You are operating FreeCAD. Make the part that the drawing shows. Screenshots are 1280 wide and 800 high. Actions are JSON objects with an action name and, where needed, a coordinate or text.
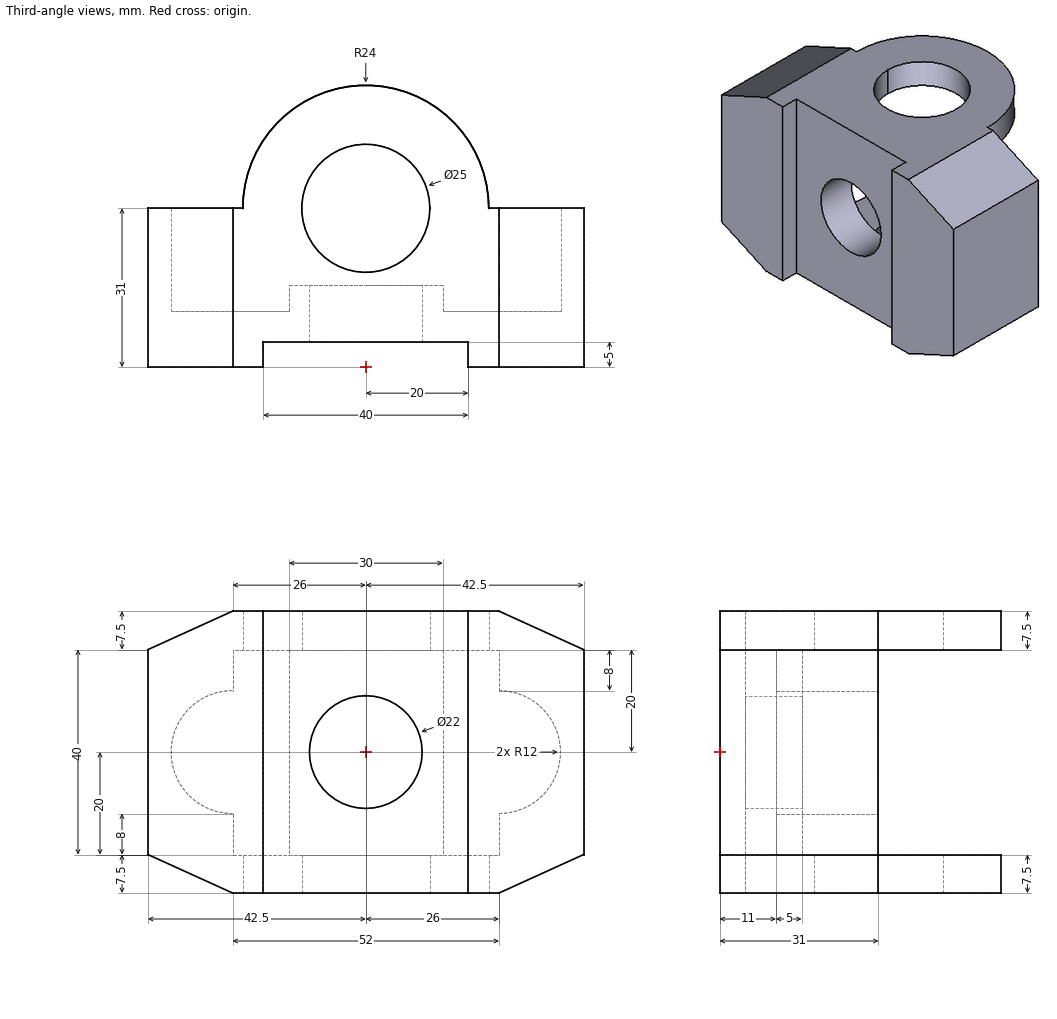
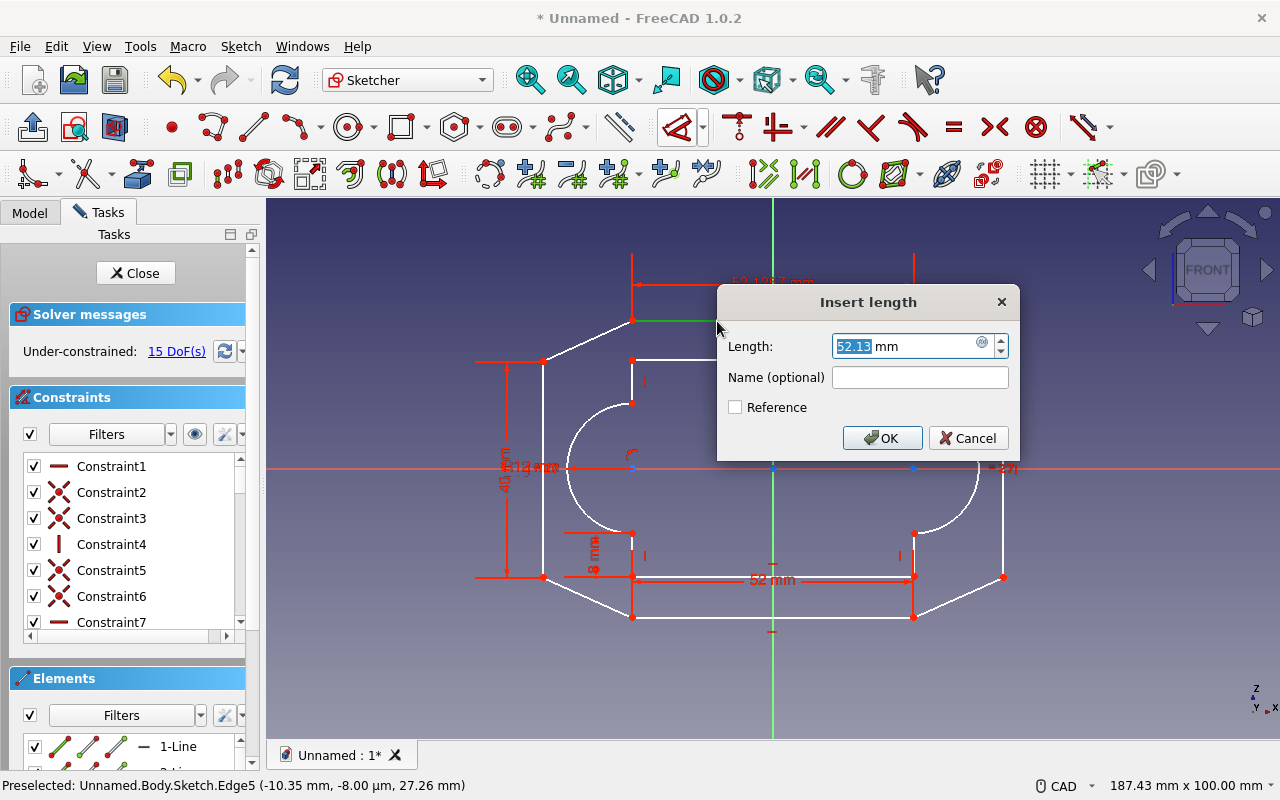
{"action": "type", "text": "52"}
{"action": "key", "text": "Return"}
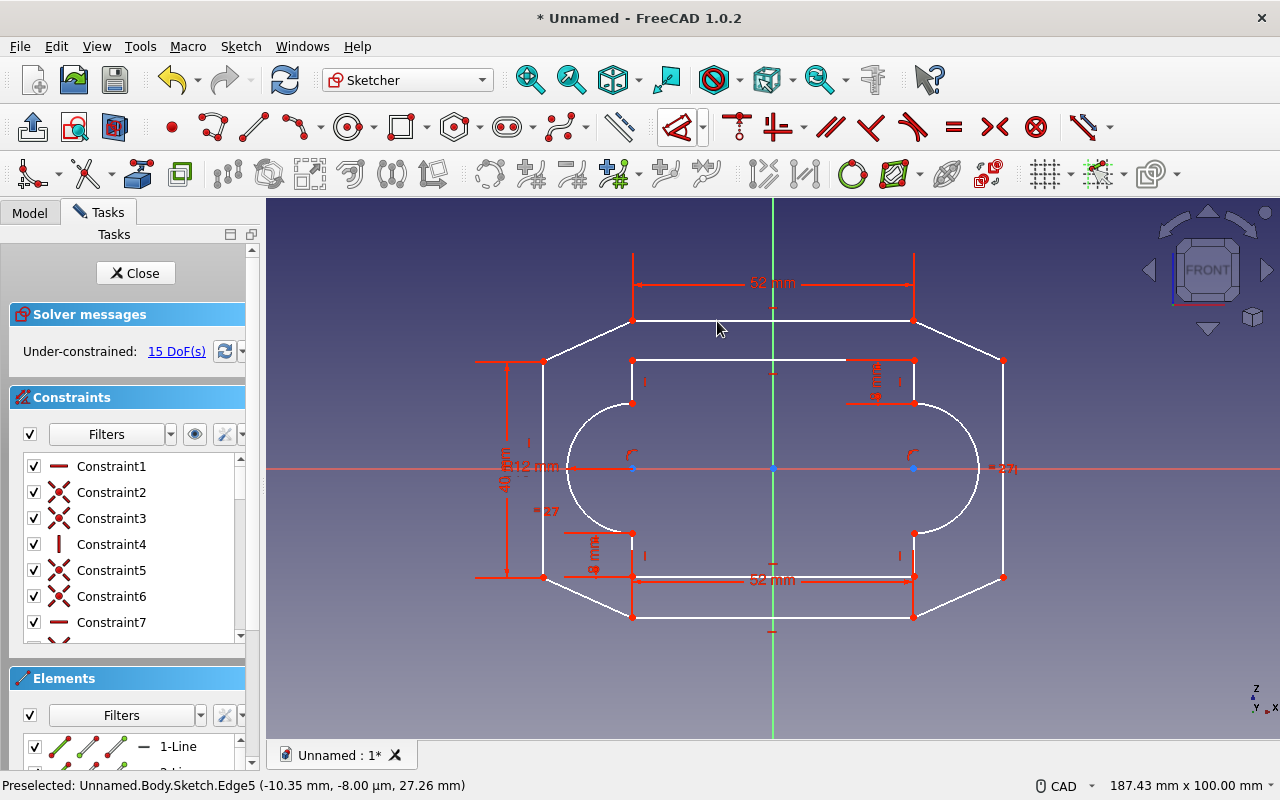
{"action": "left_click", "coordinate": [1003, 426]}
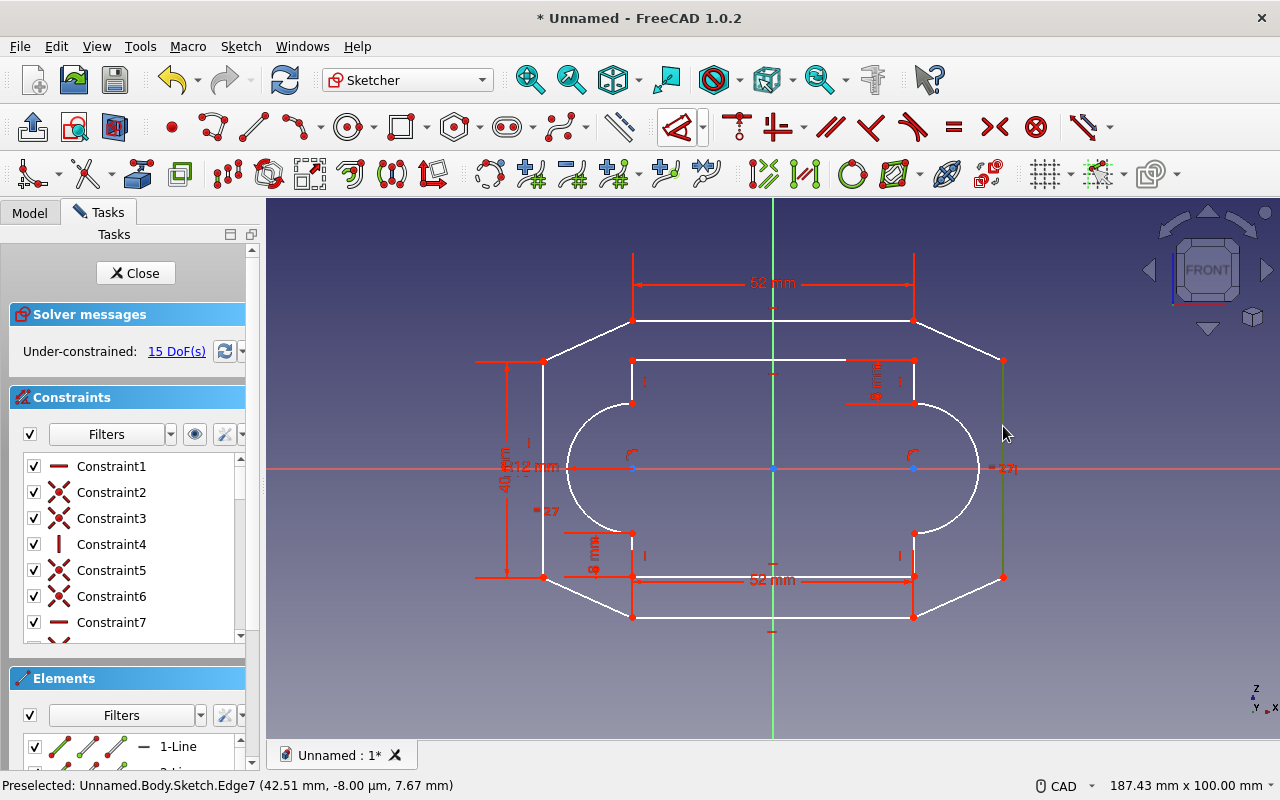
{"action": "key", "text": "i"}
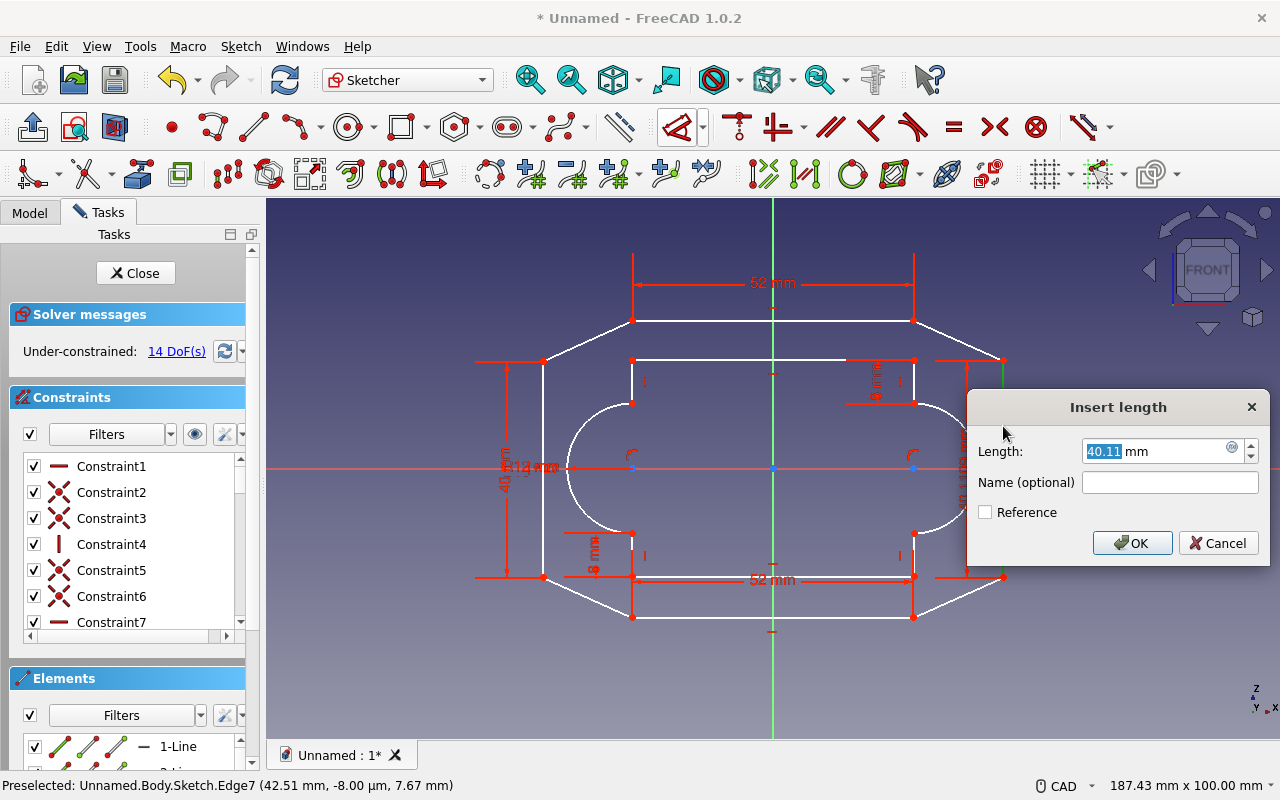
{"action": "type", "text": "40"}
{"action": "key", "text": "Return"}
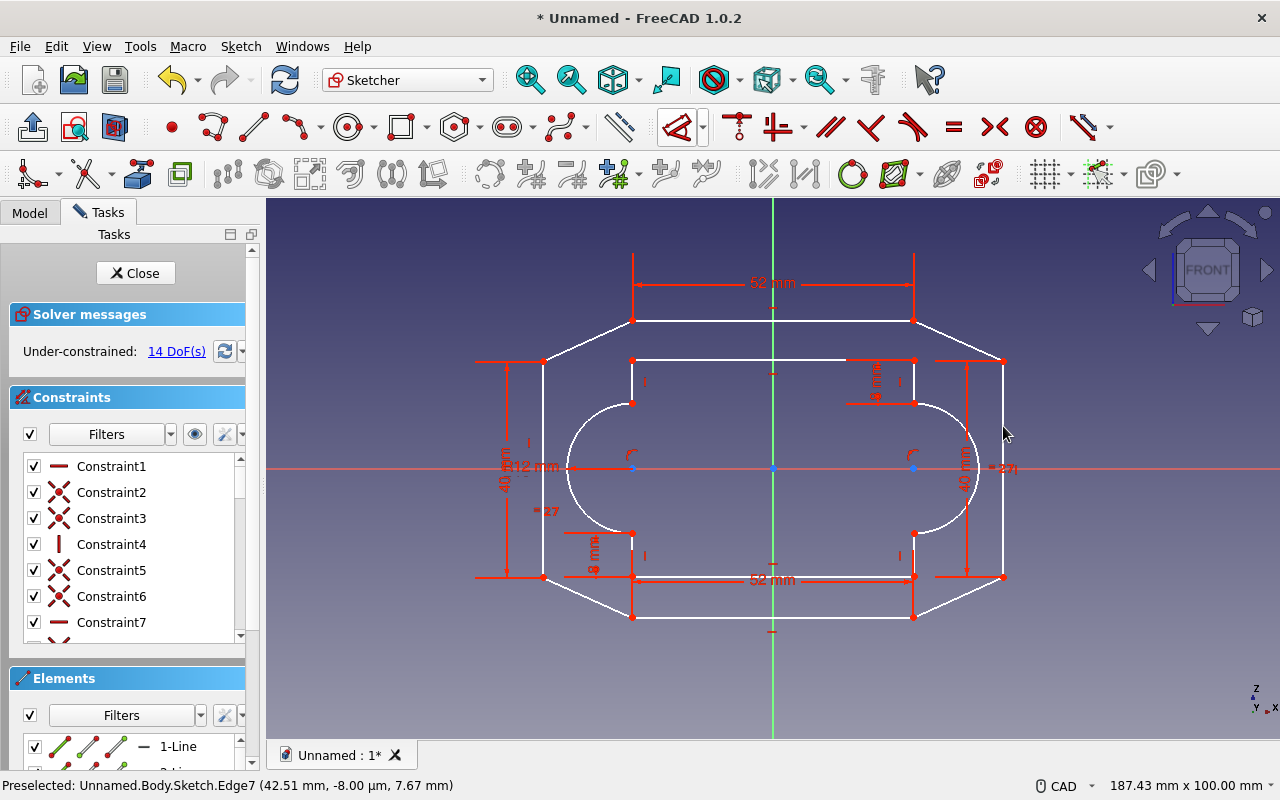
{"action": "left_click", "coordinate": [829, 360]}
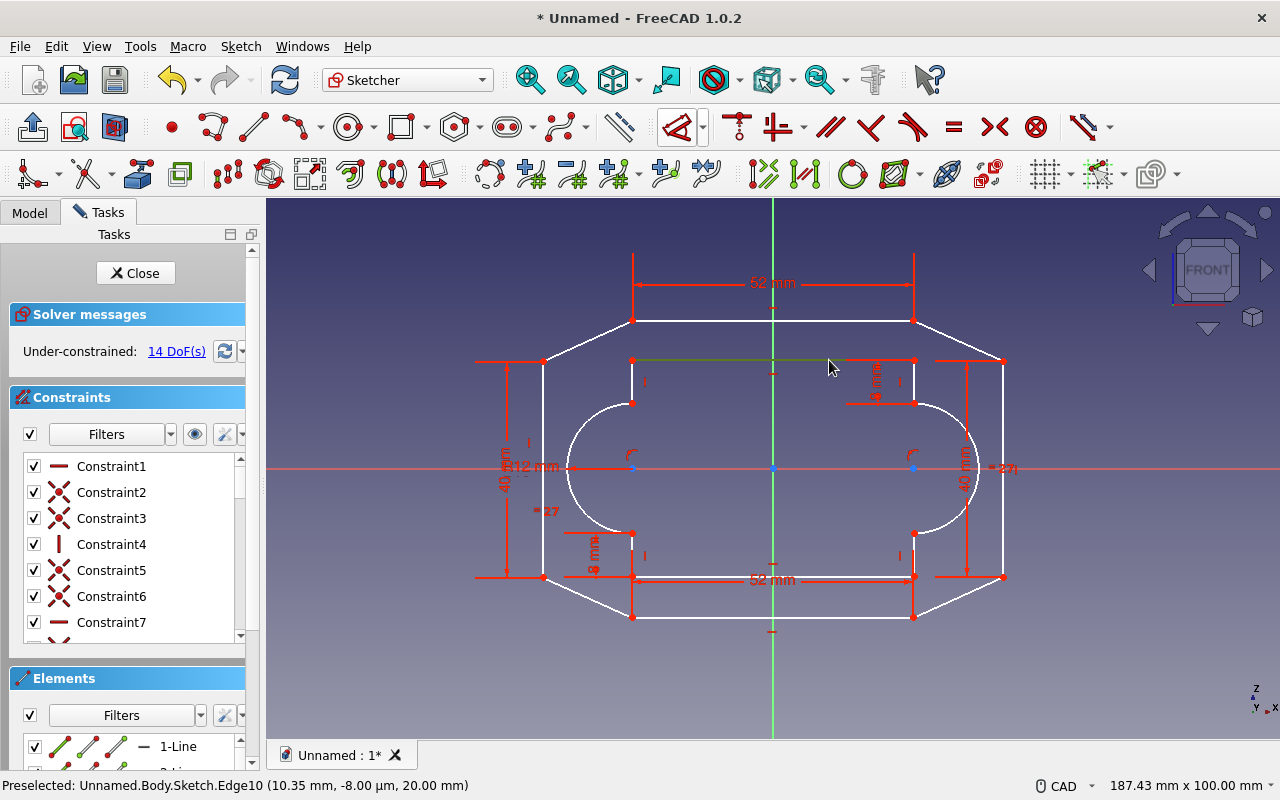
{"action": "left_click", "coordinate": [702, 128]}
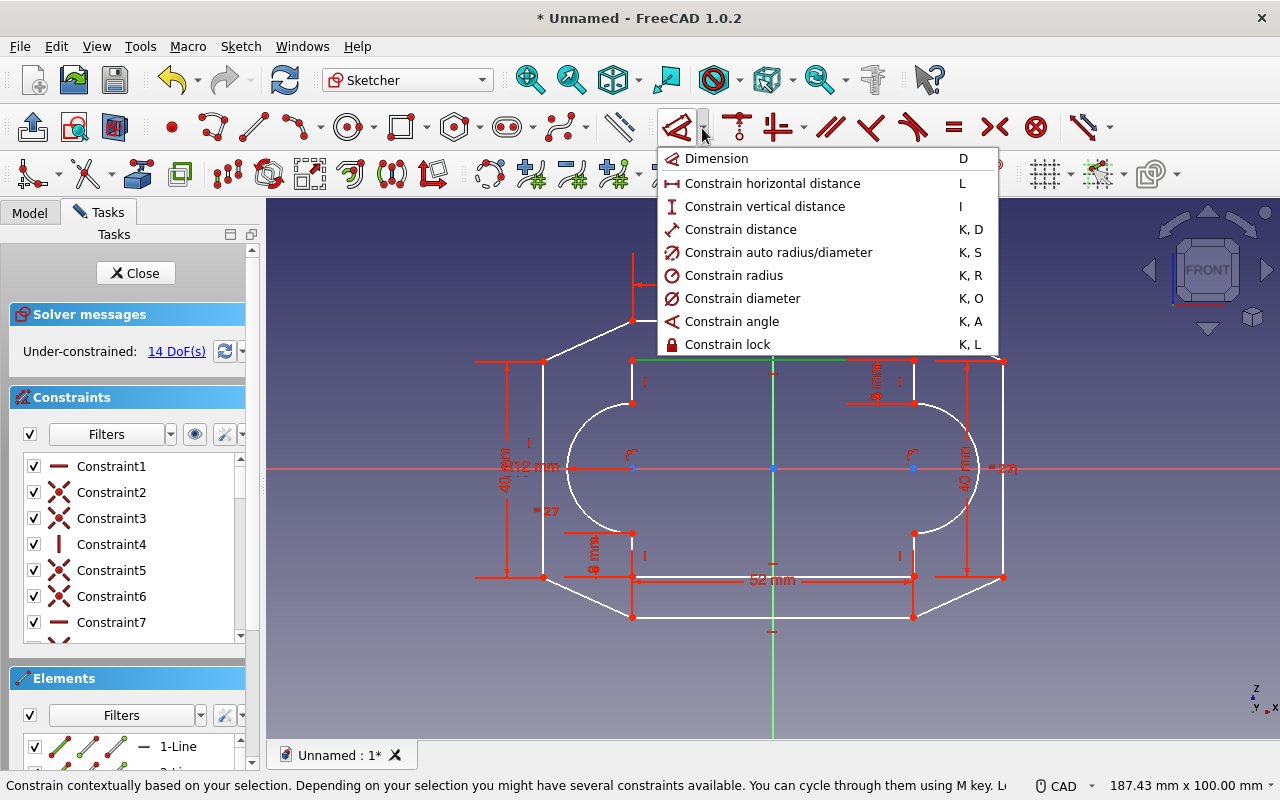
{"action": "left_click", "coordinate": [828, 184]}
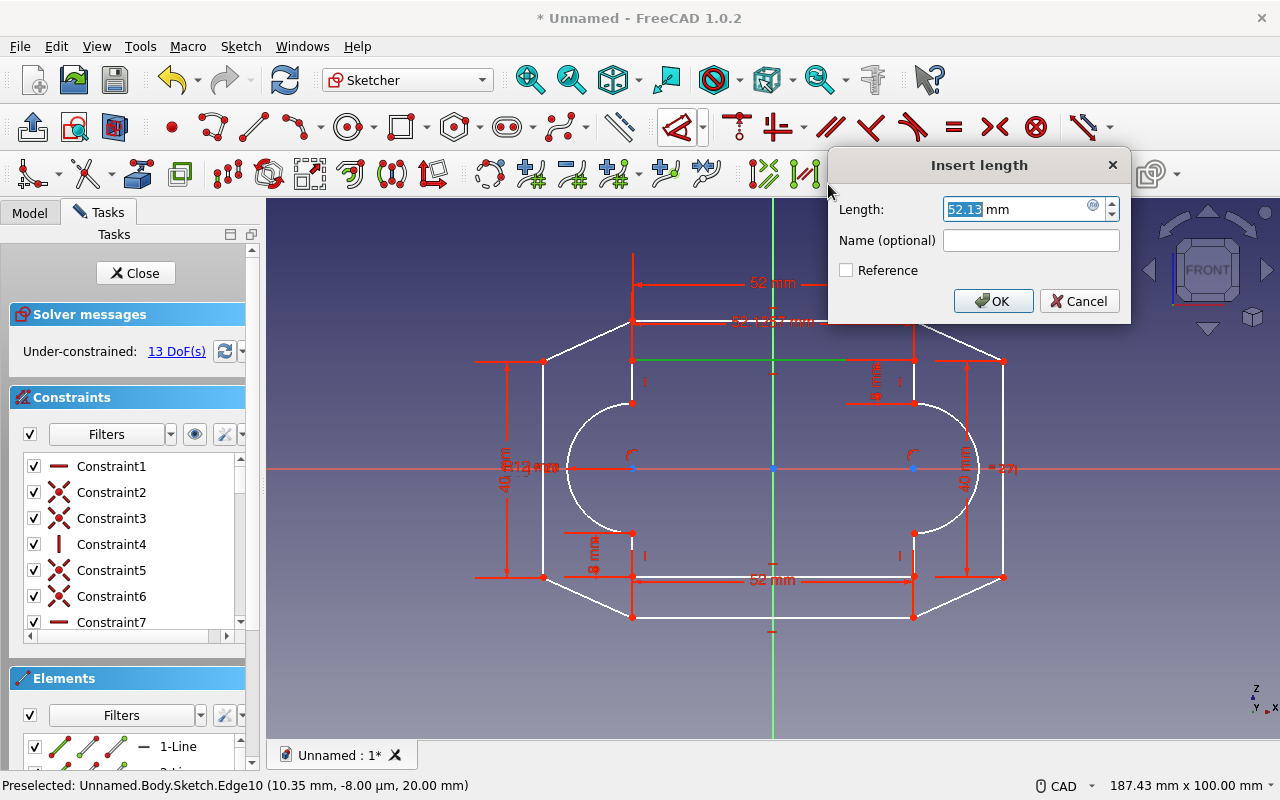
{"action": "type", "text": "52"}
{"action": "key", "text": "Return"}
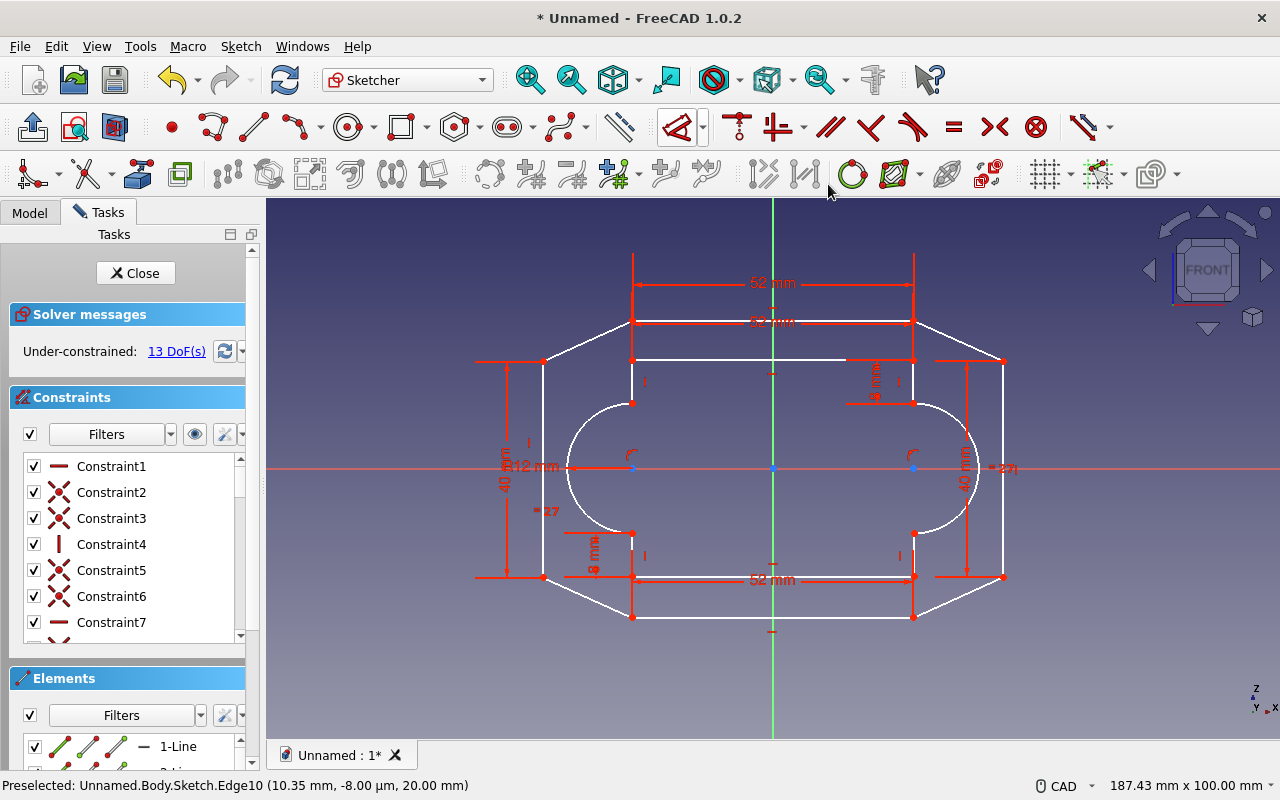
{"action": "left_click", "coordinate": [717, 577]}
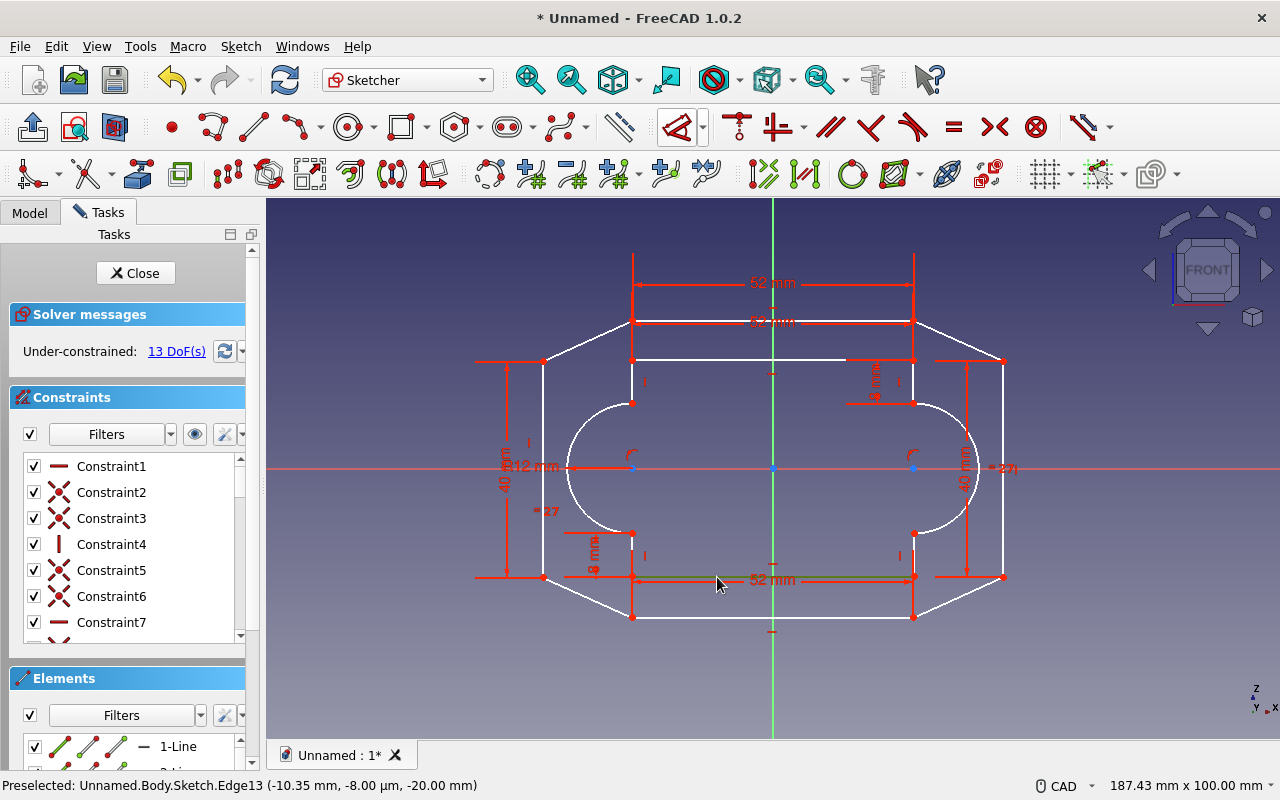
{"action": "left_click", "coordinate": [702, 128]}